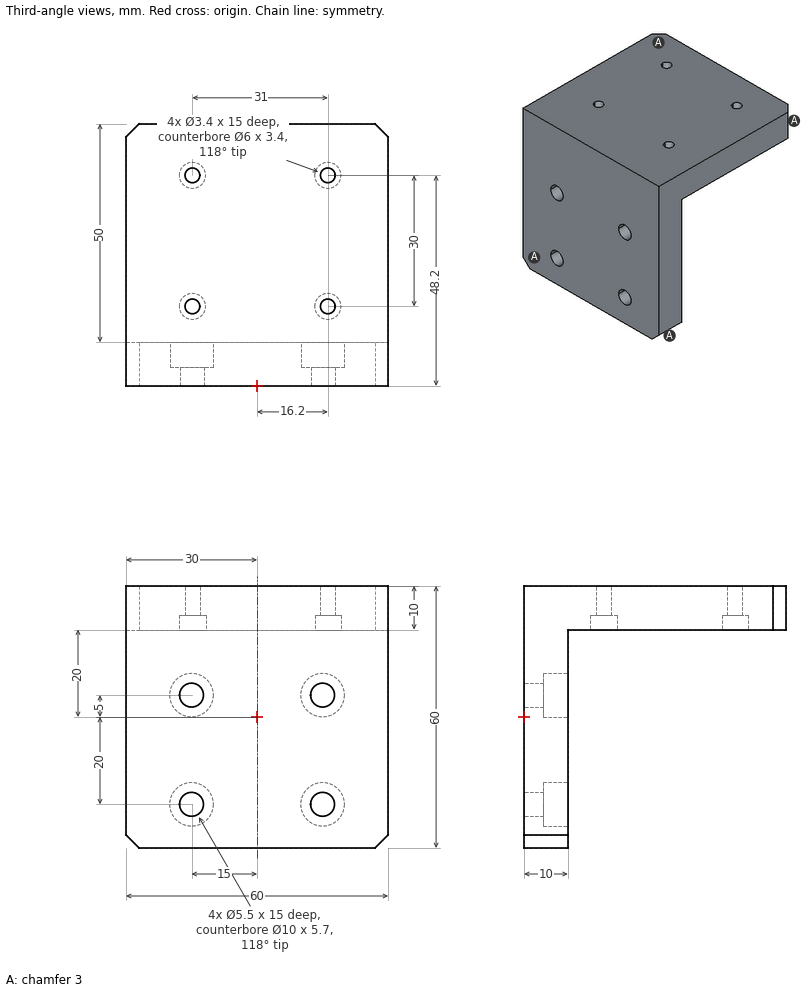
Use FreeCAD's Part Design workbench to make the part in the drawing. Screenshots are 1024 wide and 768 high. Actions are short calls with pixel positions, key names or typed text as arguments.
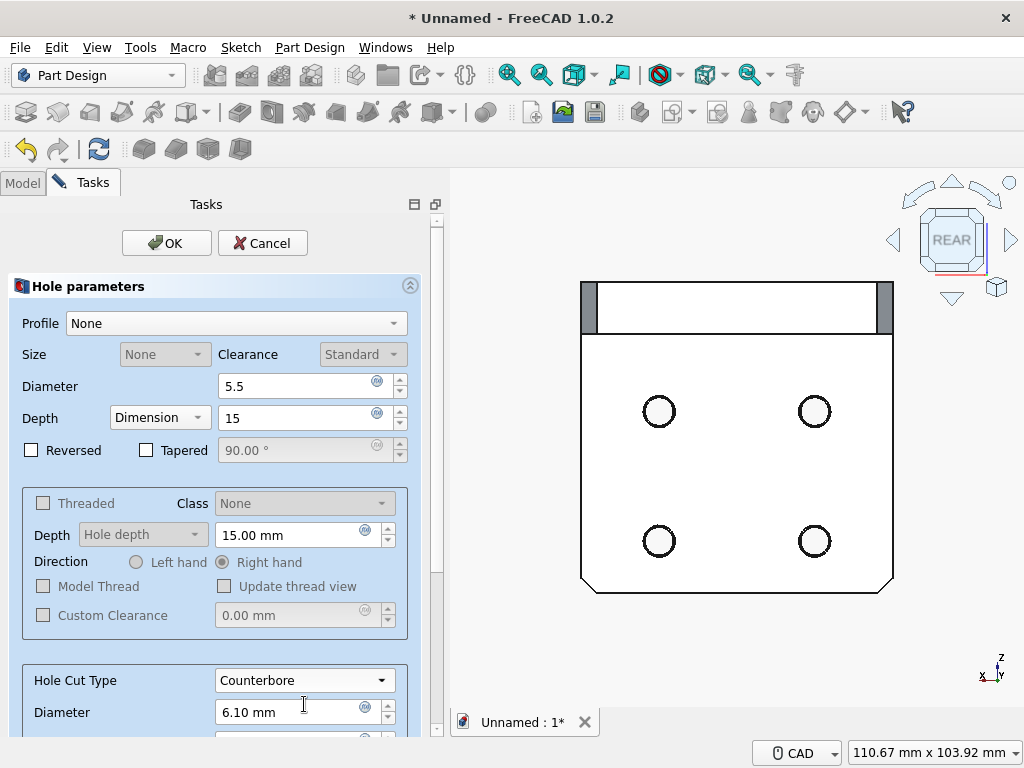
triple_click(298, 712)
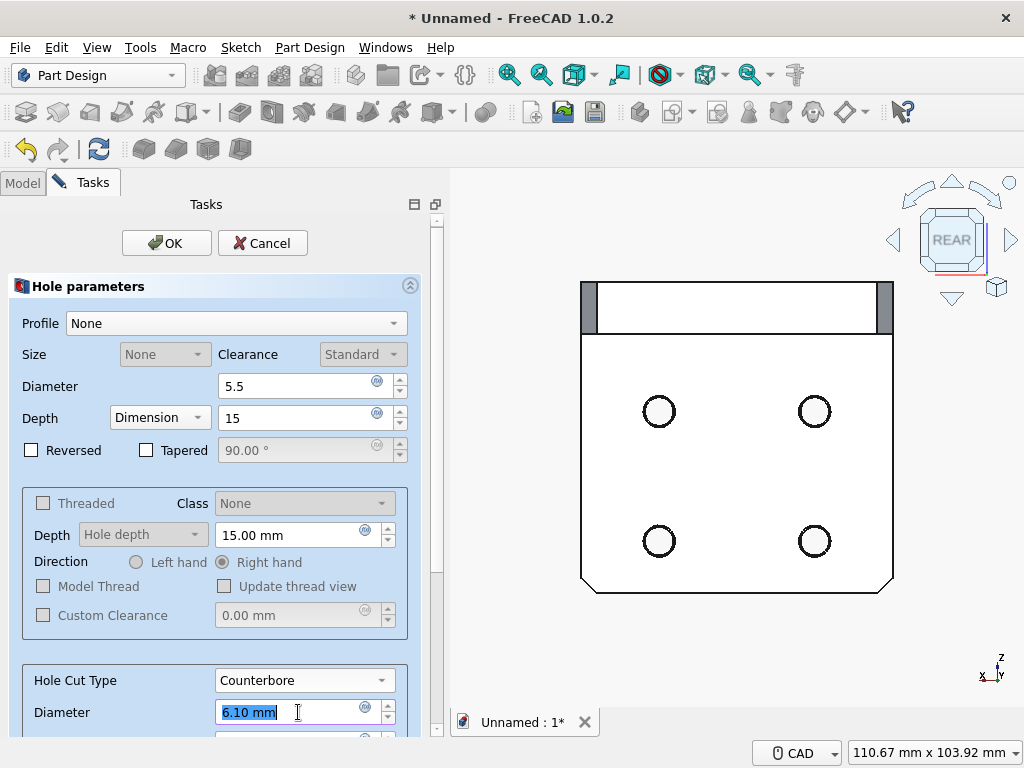
text(10)
key(Tab)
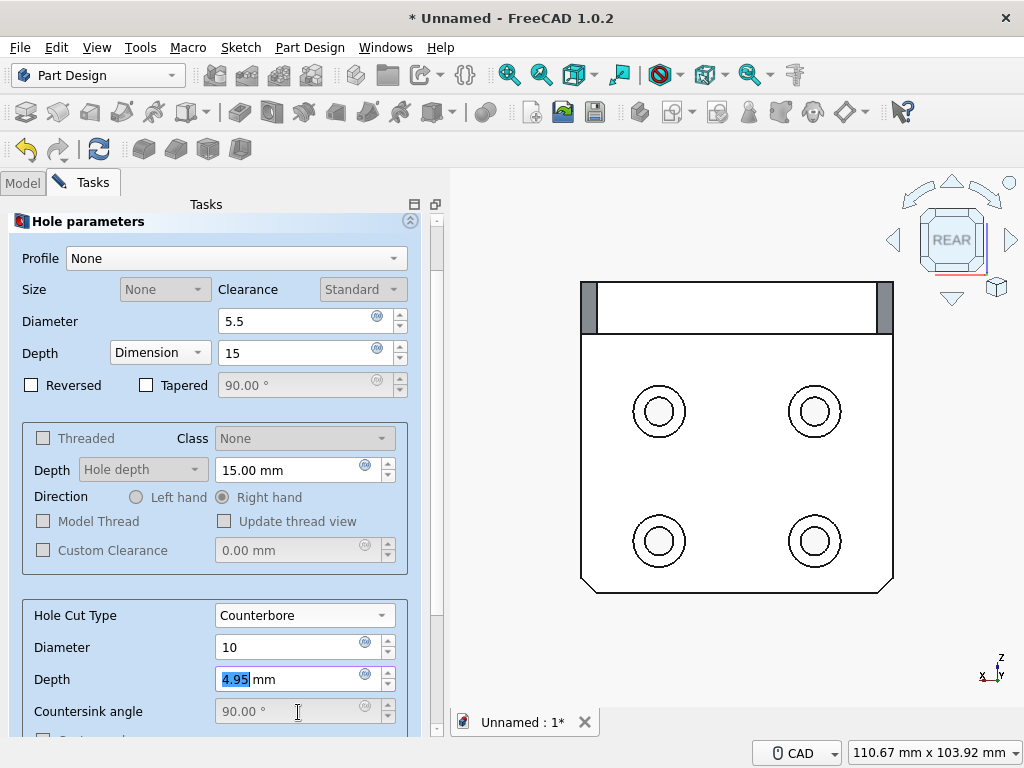
text(5.7)
key(Tab)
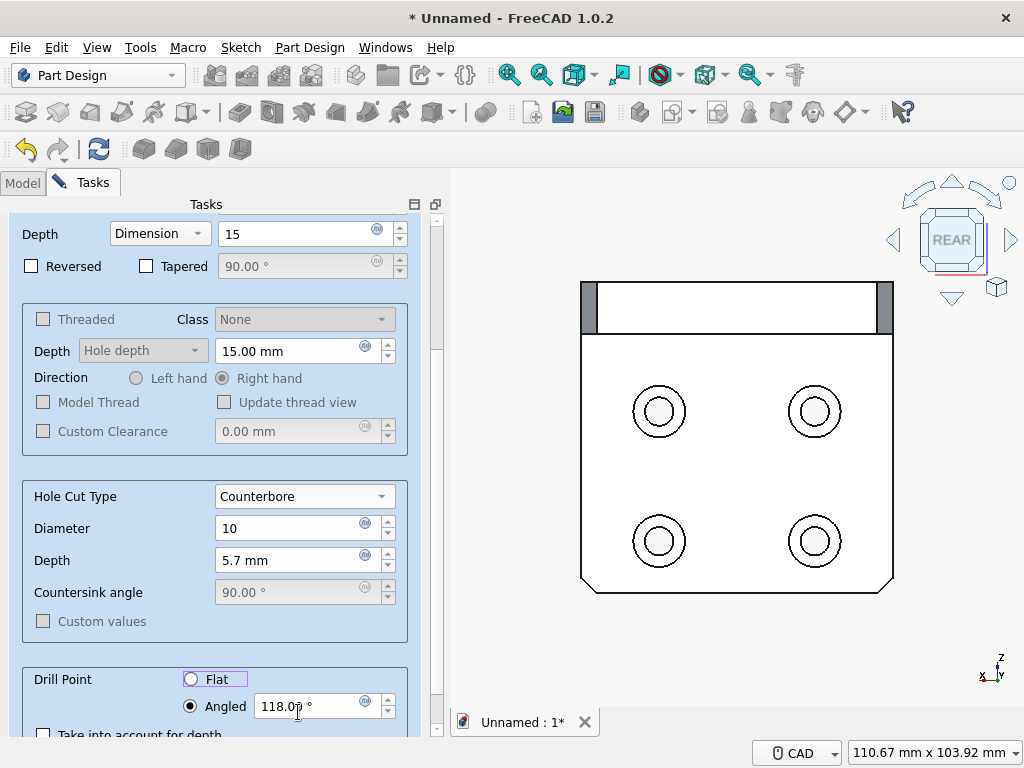
scroll(437, 475, up, 4)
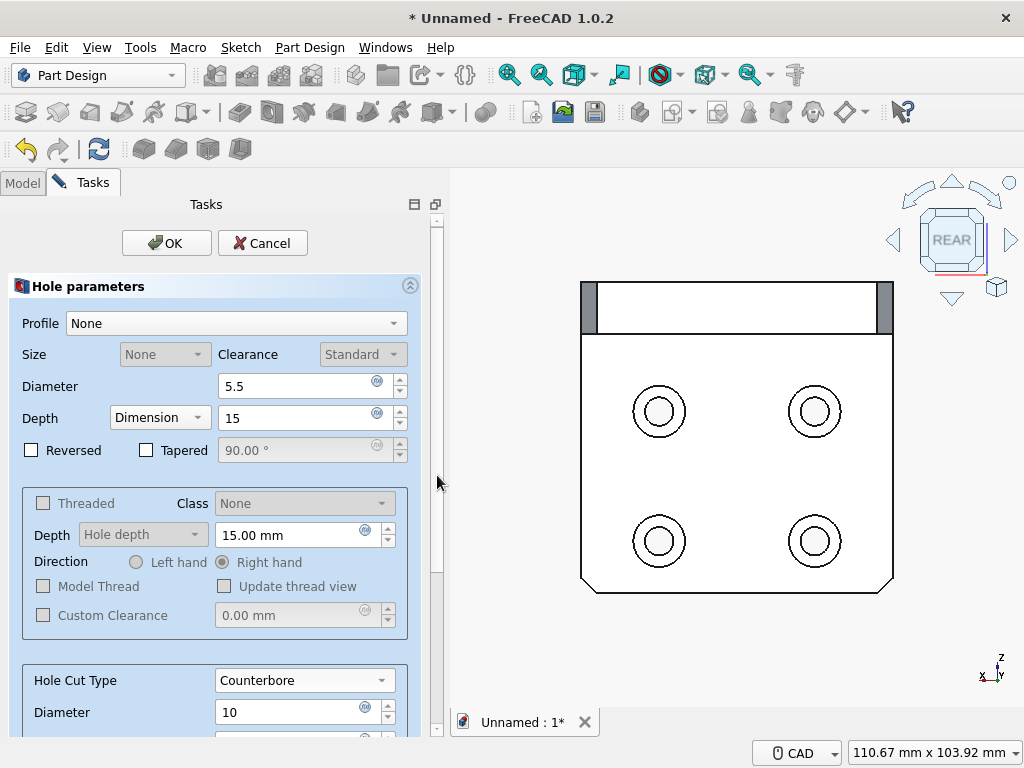
click(167, 243)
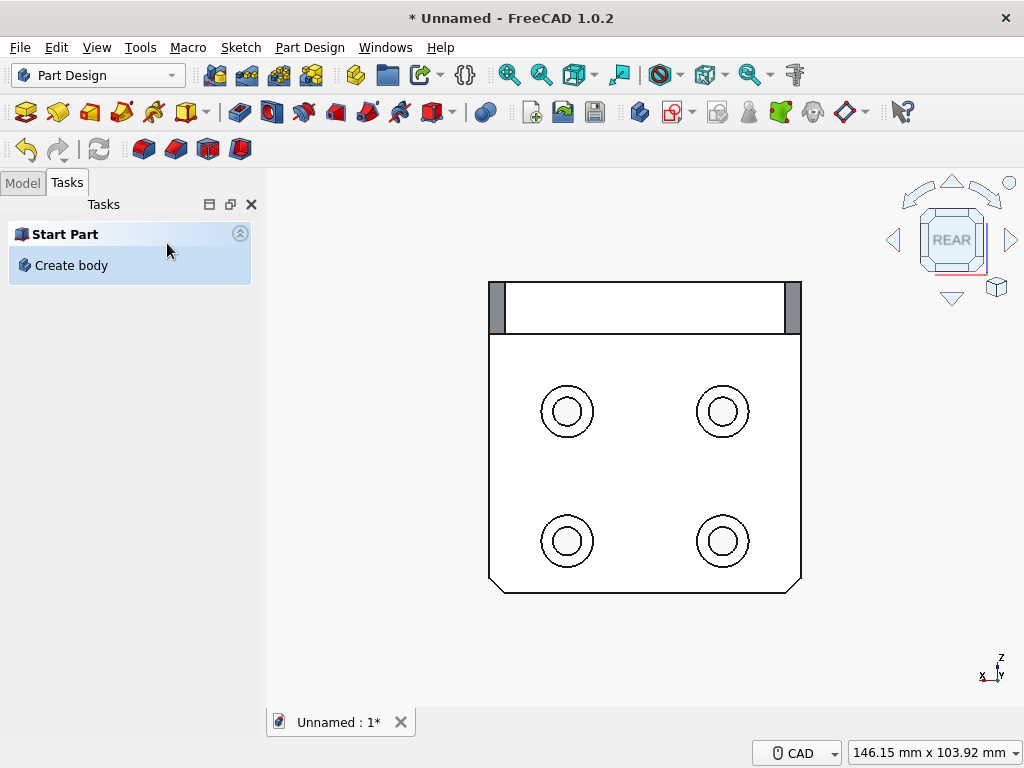
key(5)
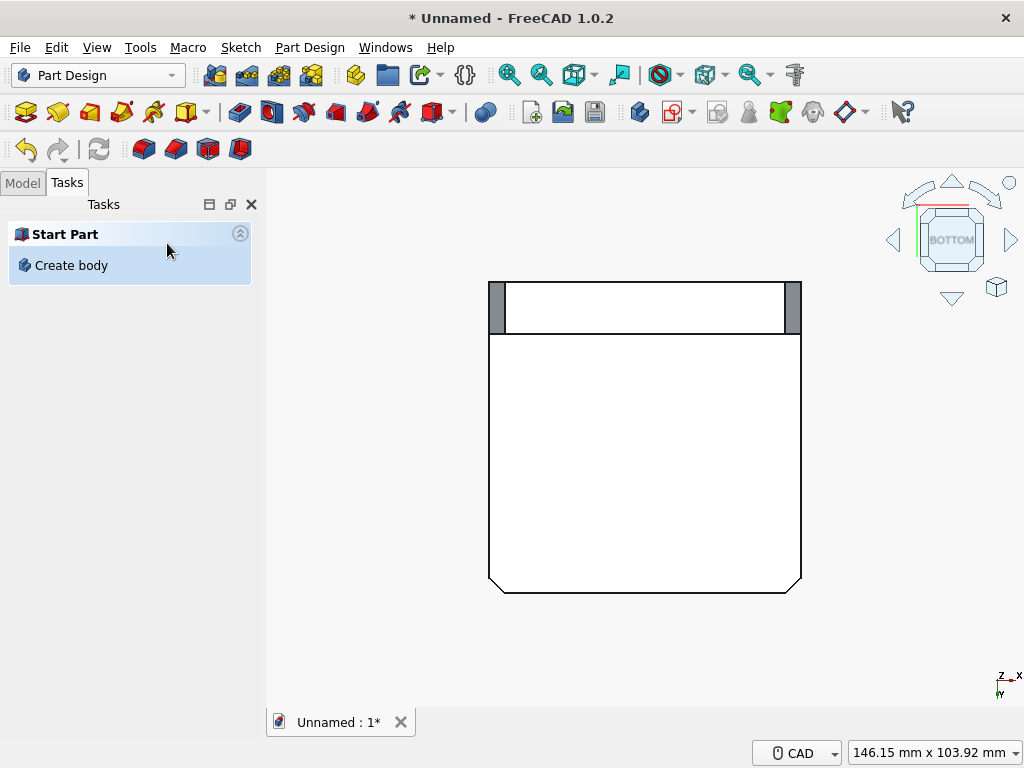
click(645, 462)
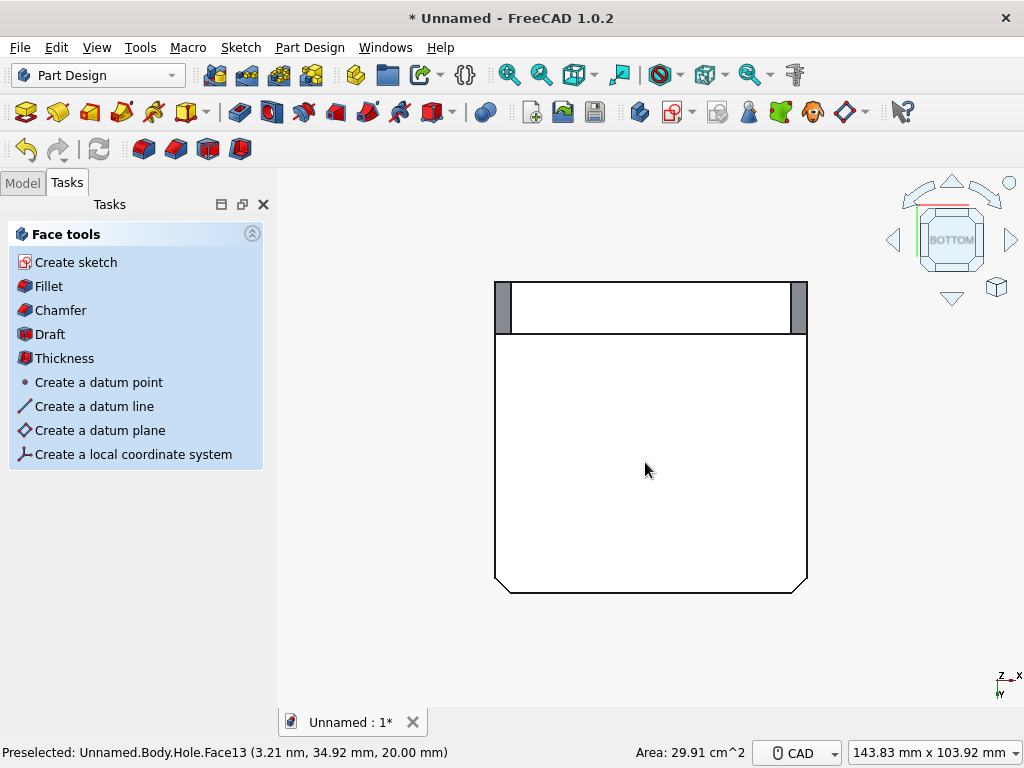
click(672, 112)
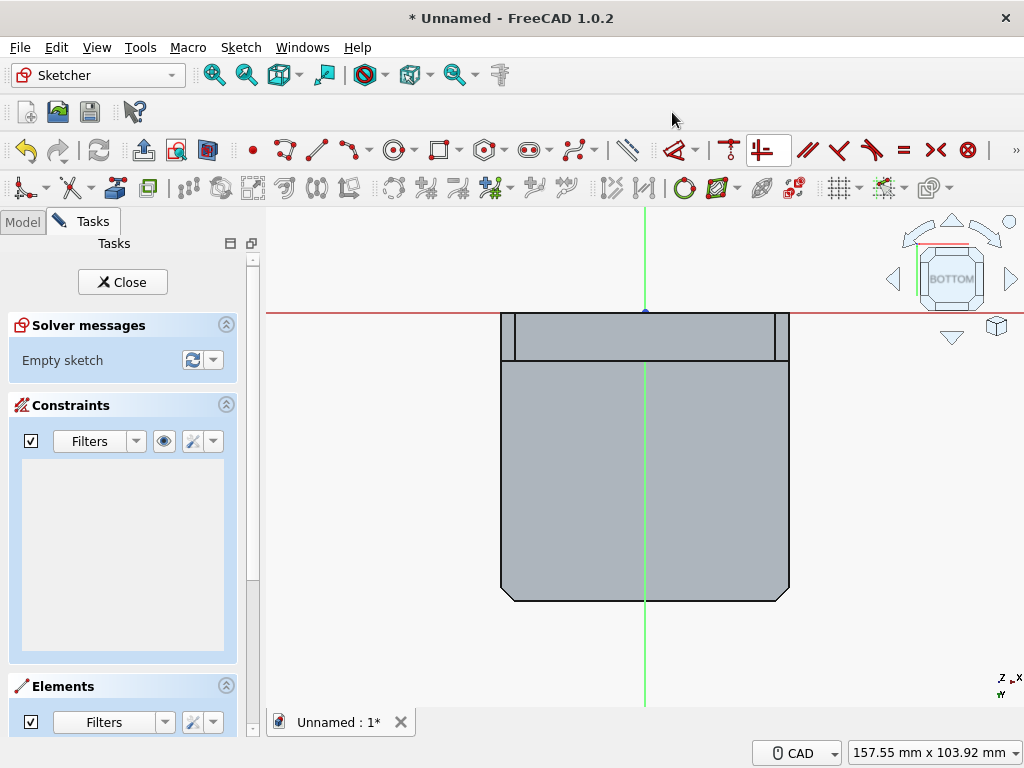
click(394, 150)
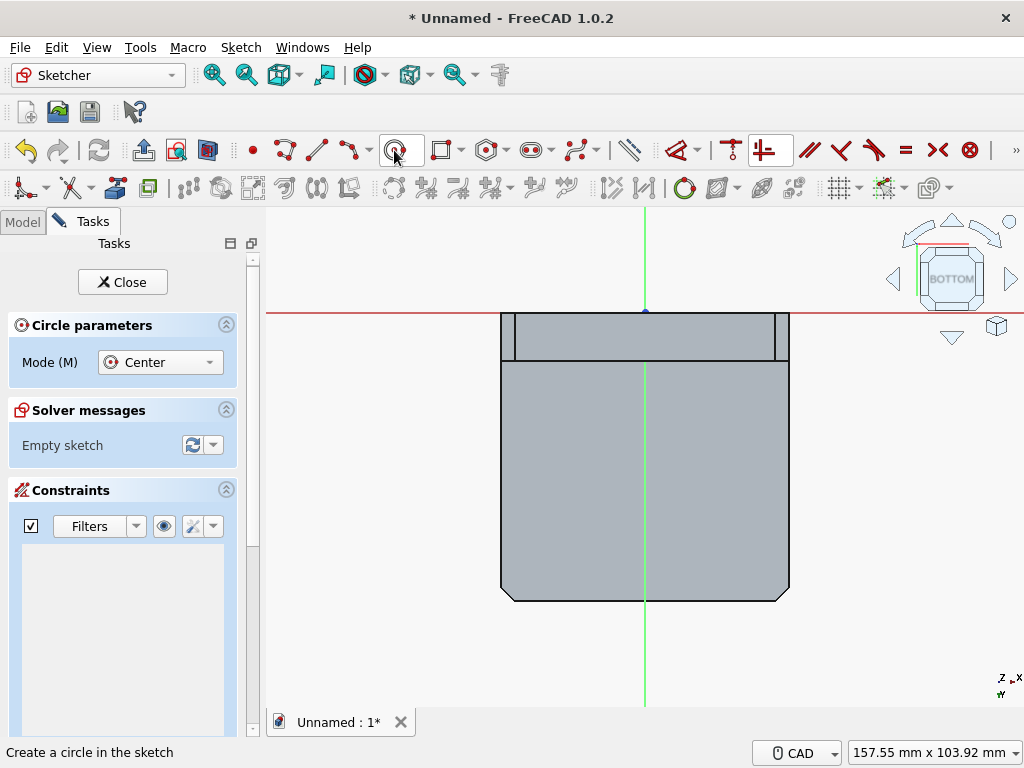
scroll(723, 545, up, 6)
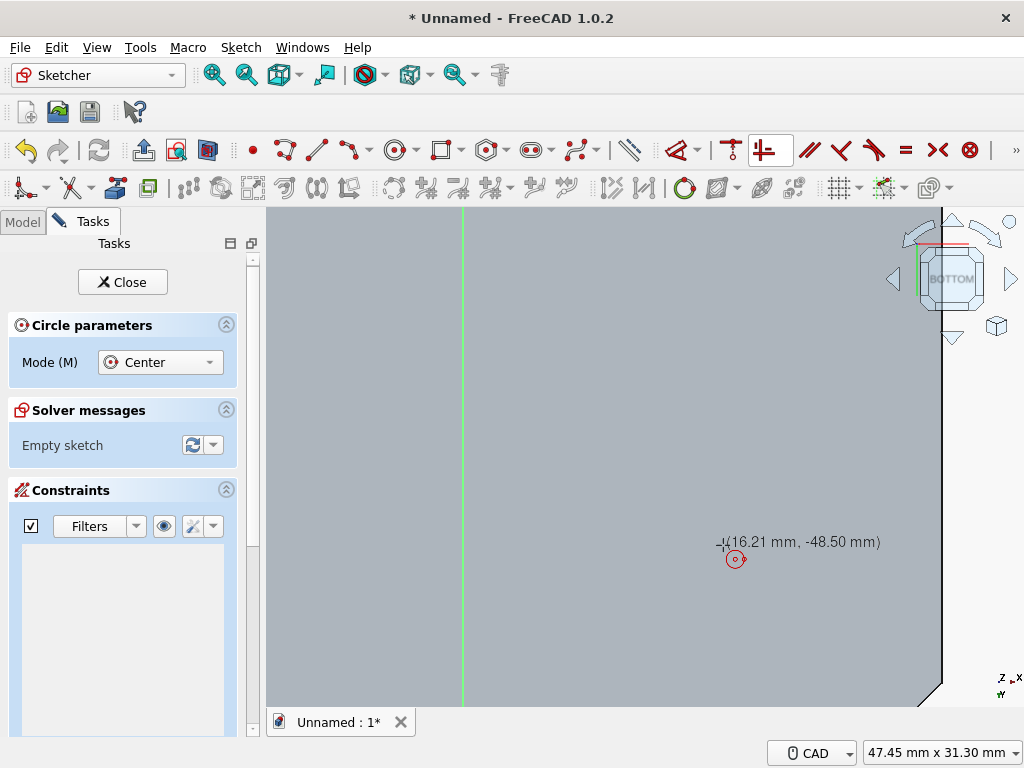
click(721, 542)
move(741, 523)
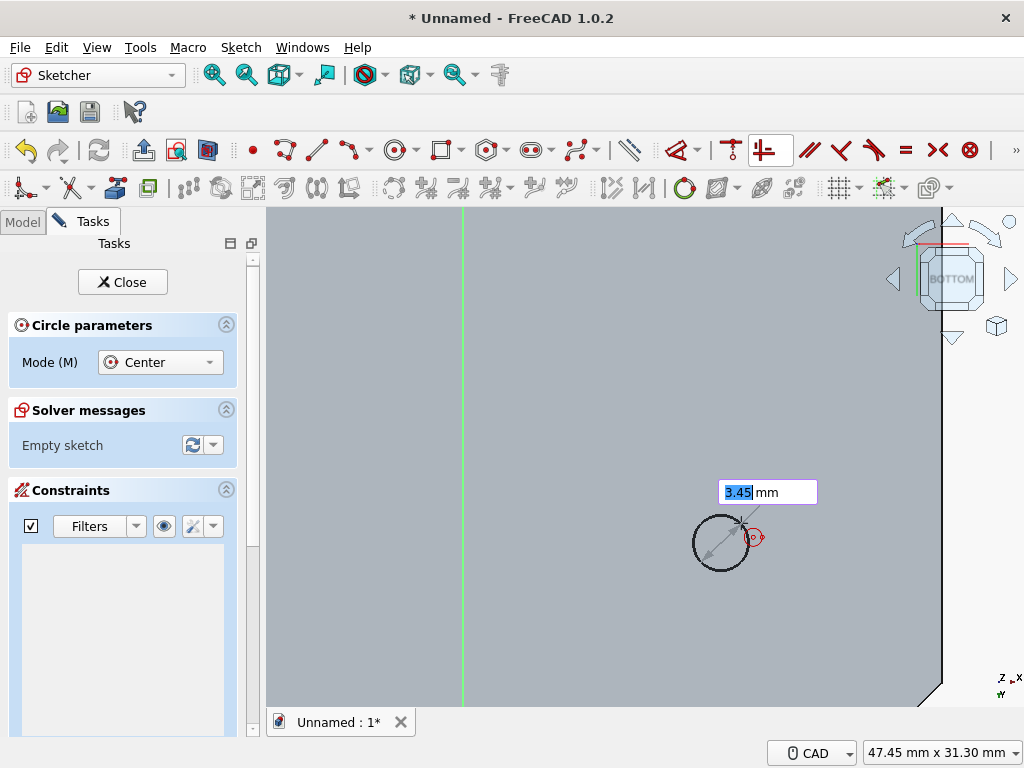
text(3.4)
key(Return)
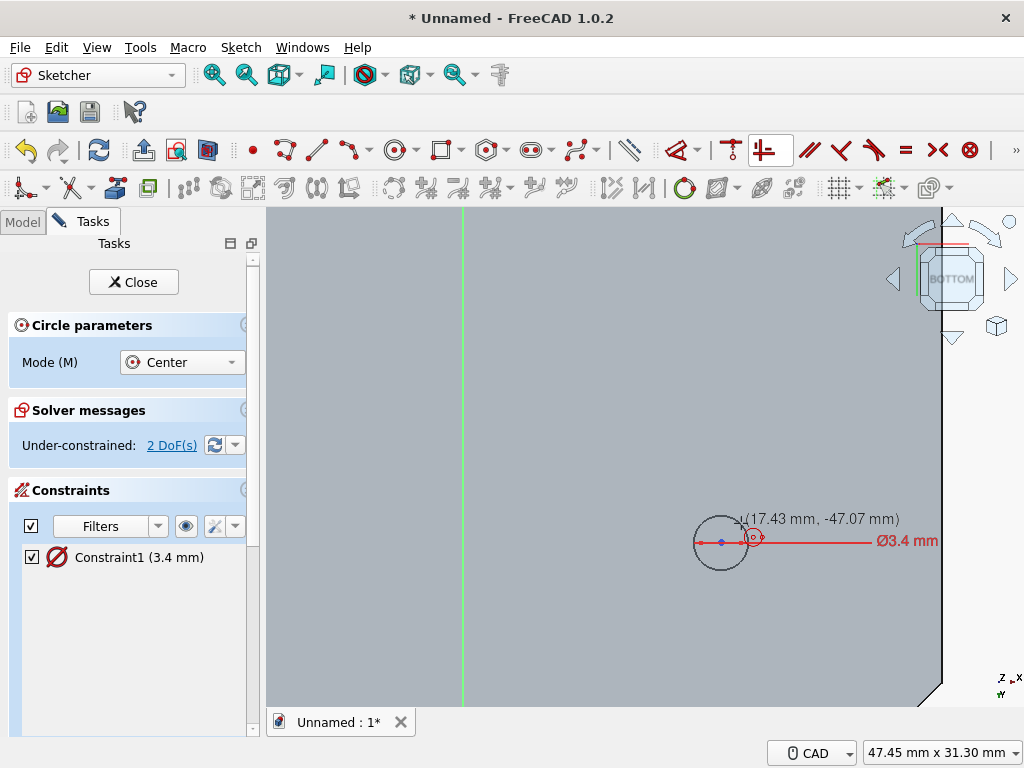
scroll(636, 624, down, 5)